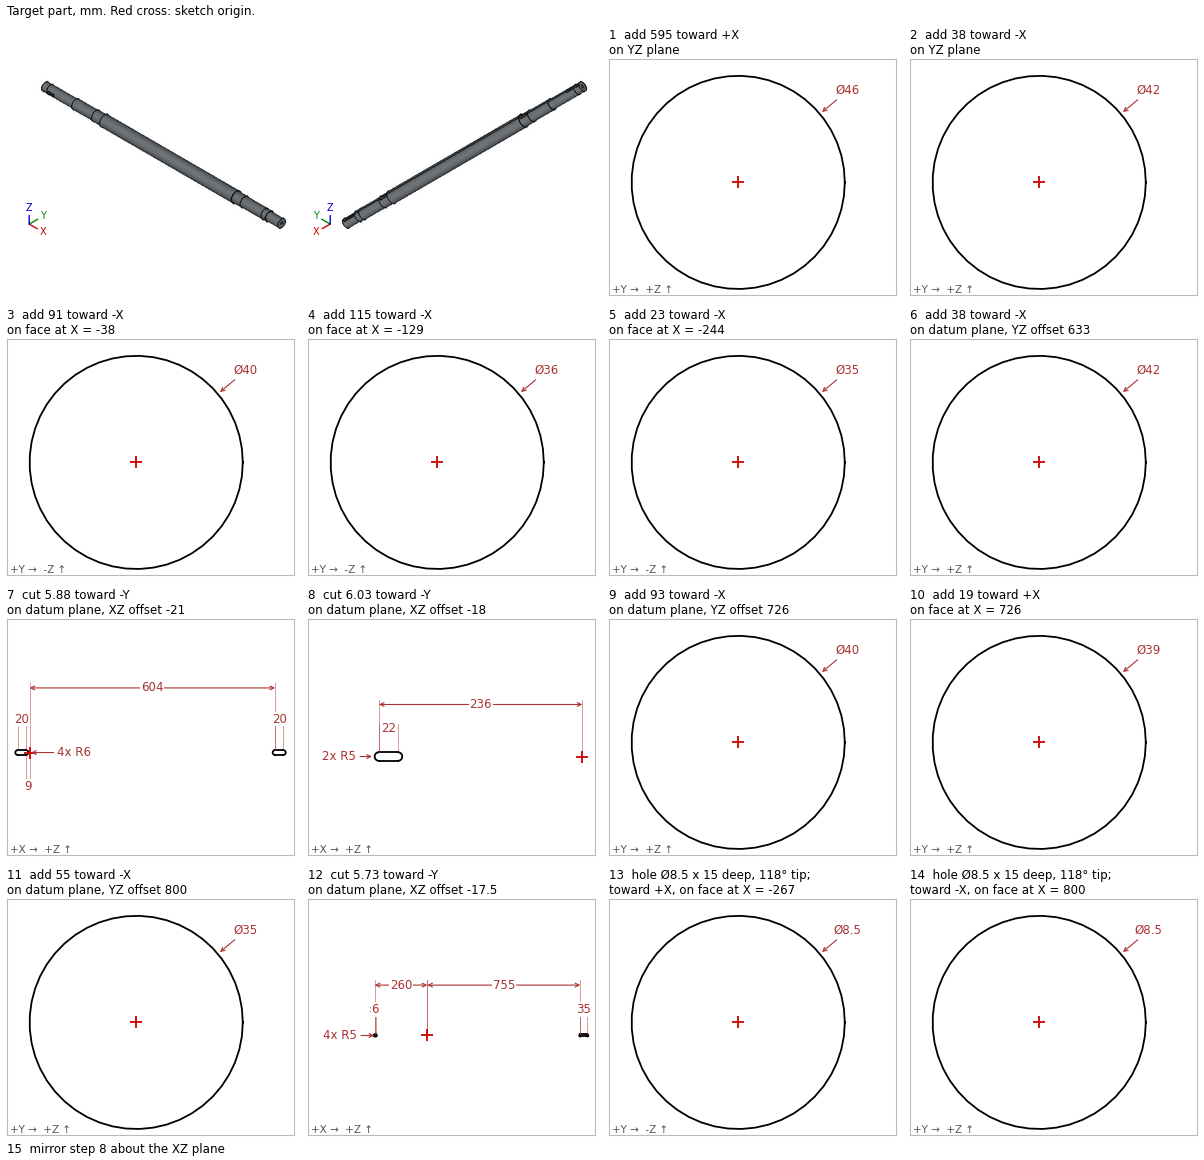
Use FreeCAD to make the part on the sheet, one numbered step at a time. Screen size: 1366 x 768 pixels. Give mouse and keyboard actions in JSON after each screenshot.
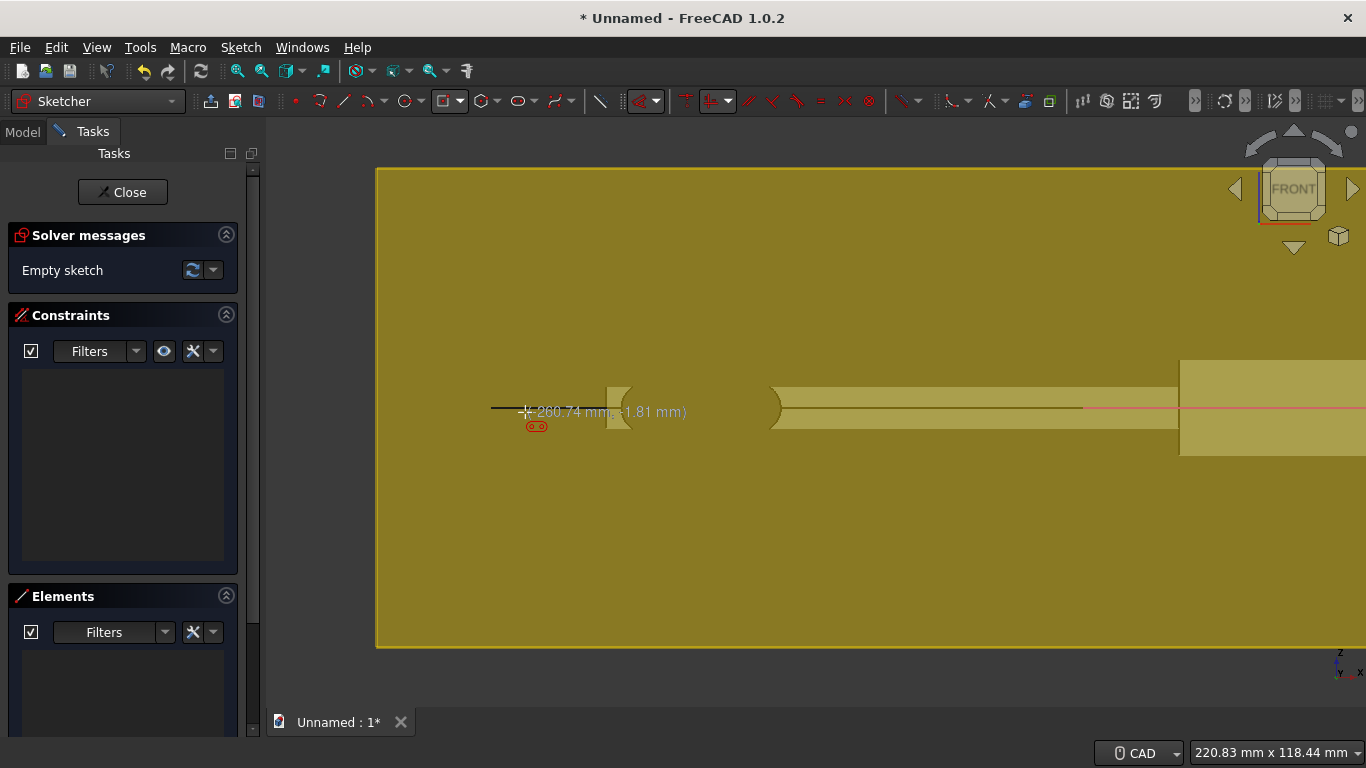
{"action": "scroll", "coordinate": [449, 413], "scroll_direction": "down", "scroll_amount": 11}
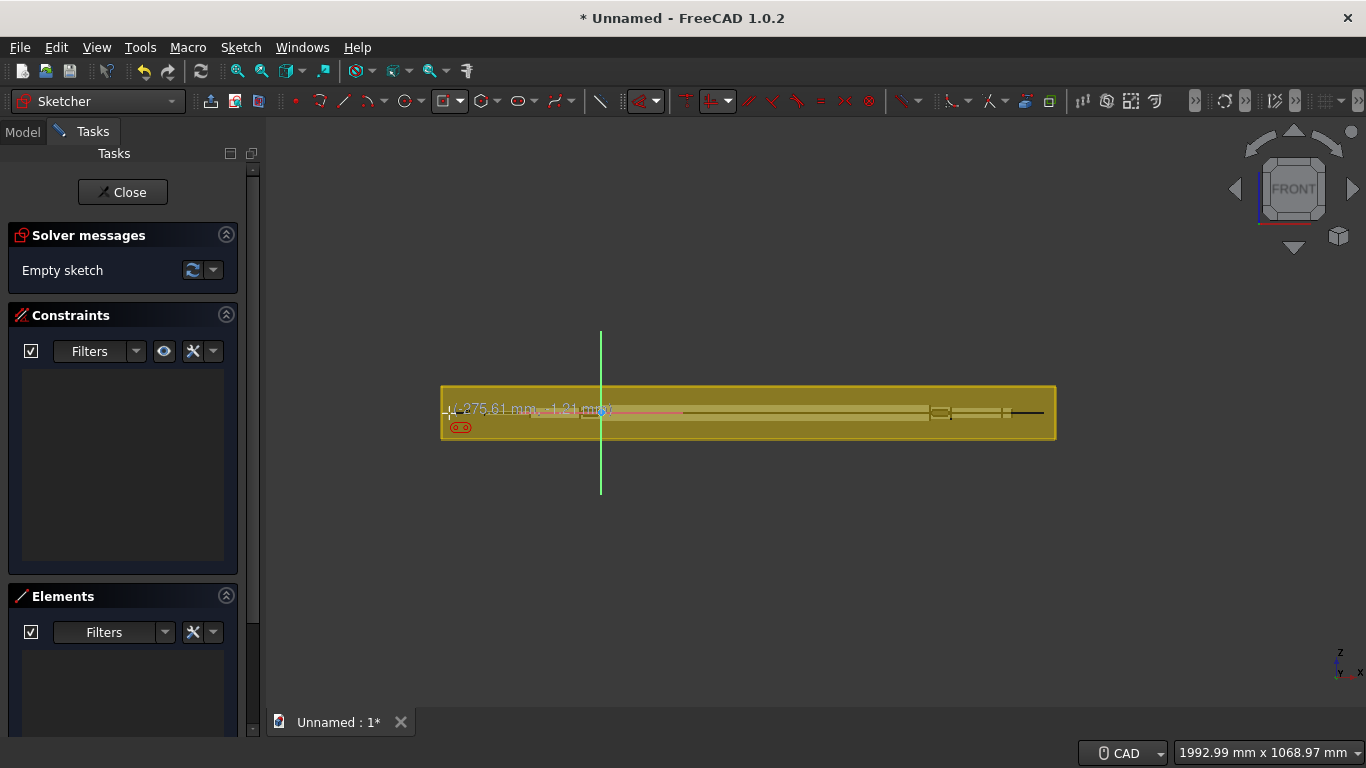
{"action": "left_click", "coordinate": [458, 413]}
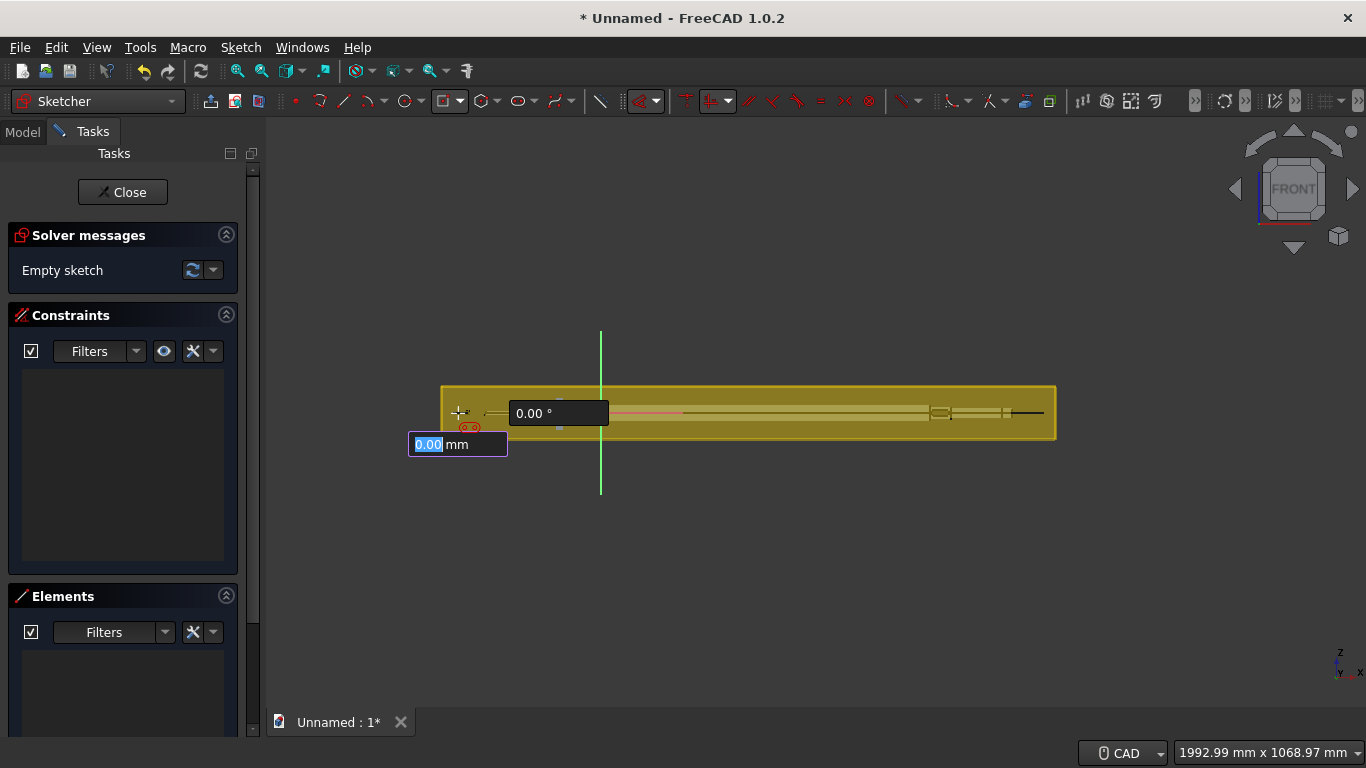
{"action": "scroll", "coordinate": [461, 413], "scroll_direction": "up", "scroll_amount": 8}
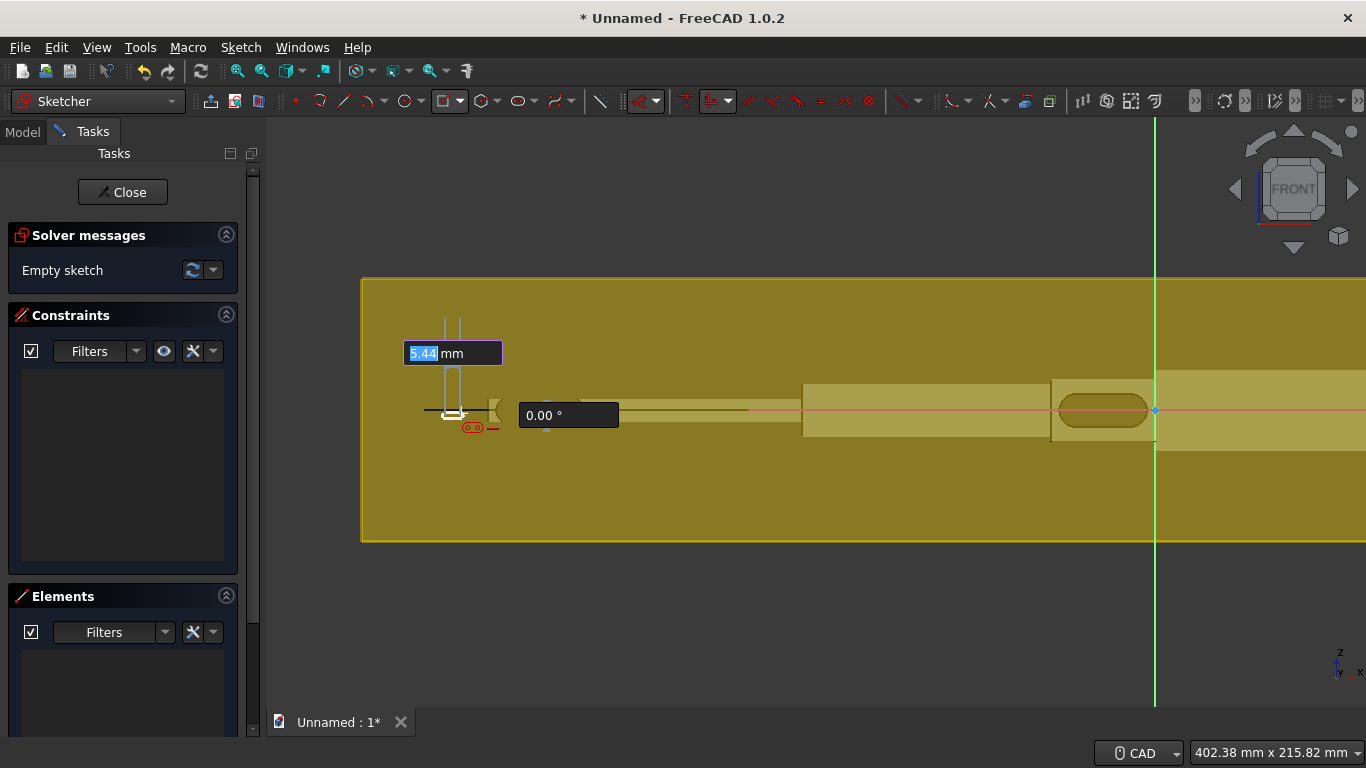
{"action": "left_click", "coordinate": [461, 401]}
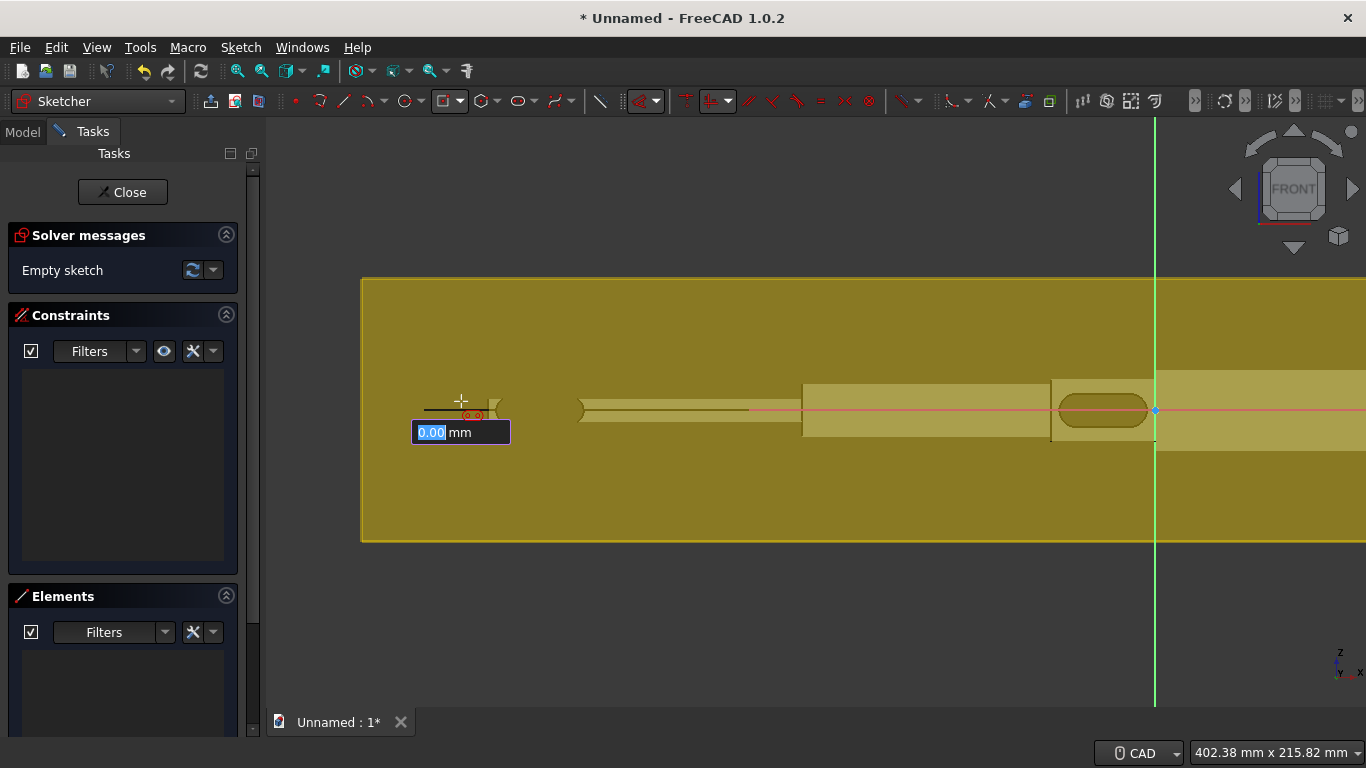
{"action": "left_click", "coordinate": [452, 397]}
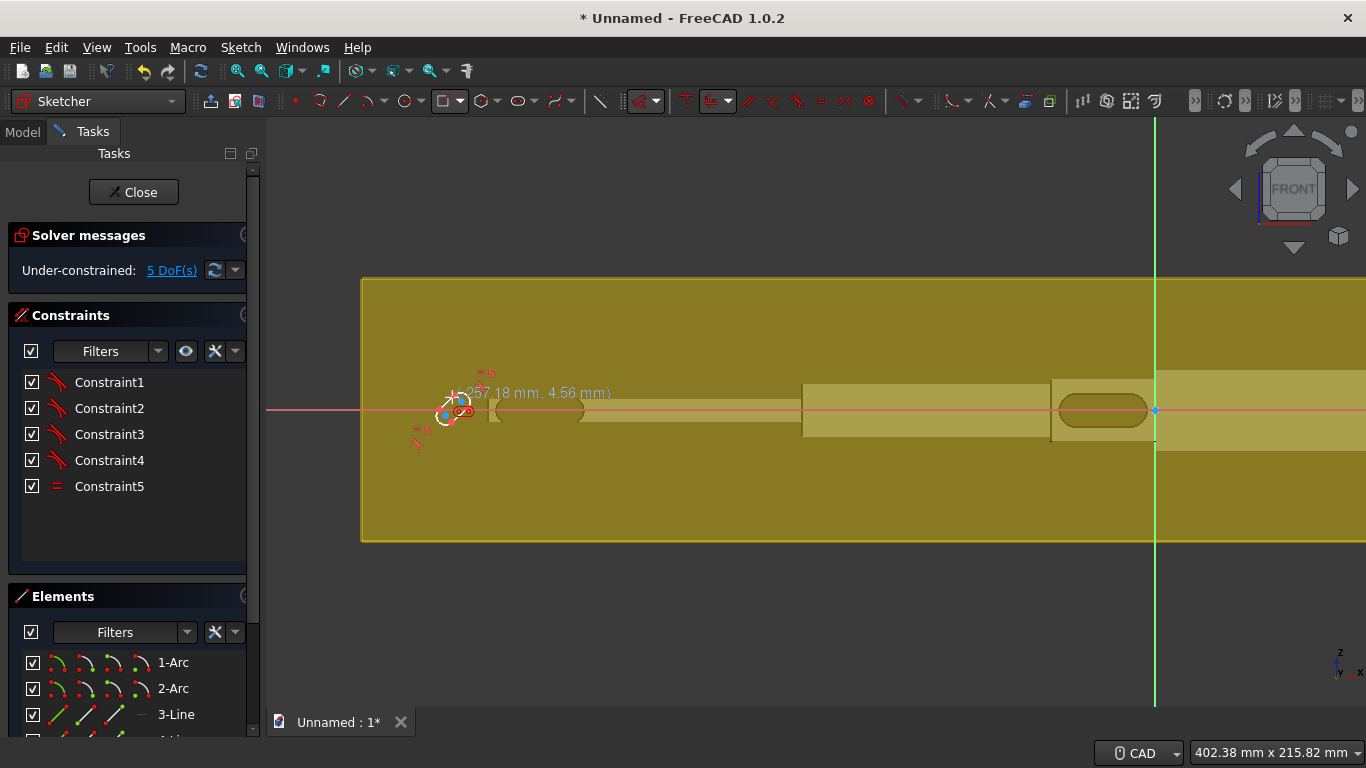
{"action": "scroll", "coordinate": [461, 412], "scroll_direction": "down", "scroll_amount": 8}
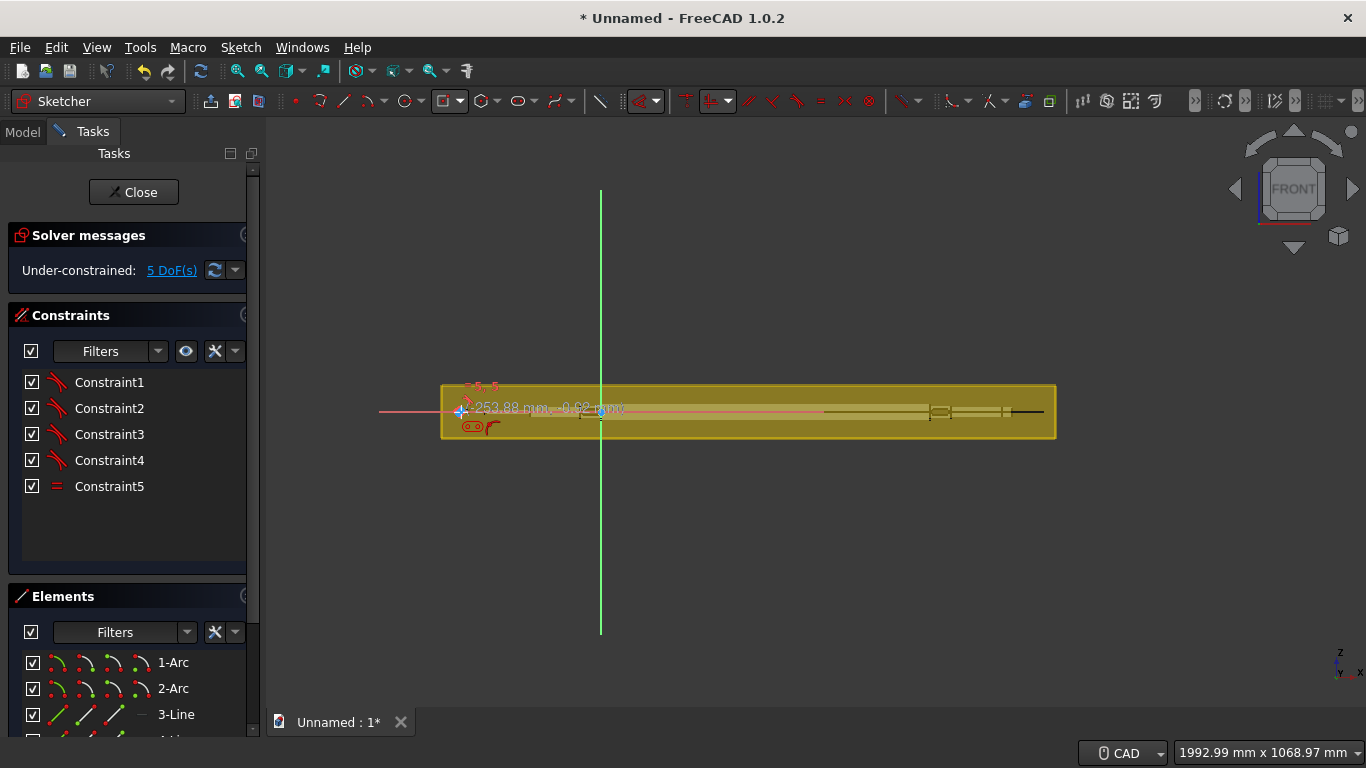
{"action": "scroll", "coordinate": [1018, 412], "scroll_direction": "up", "scroll_amount": 11}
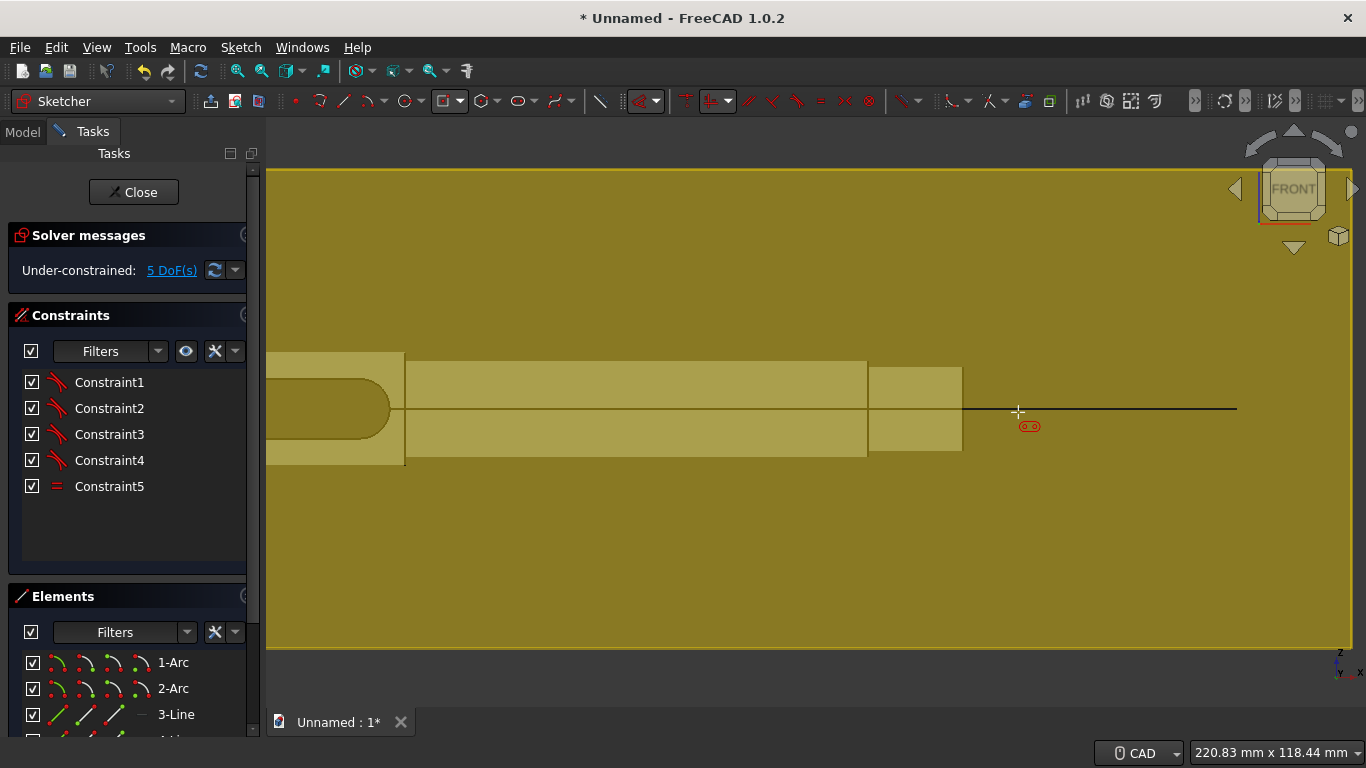
{"action": "scroll", "coordinate": [1019, 412], "scroll_direction": "down", "scroll_amount": 11}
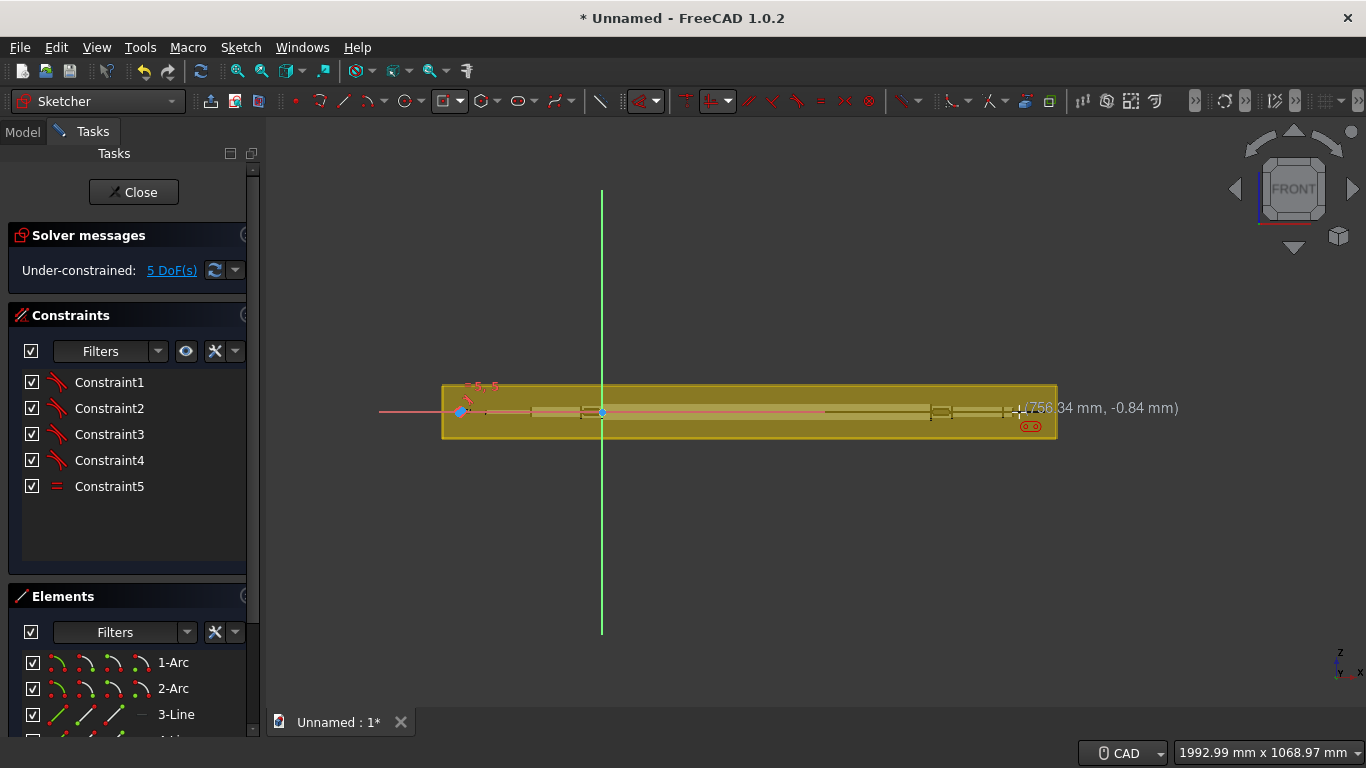
{"action": "left_click", "coordinate": [1019, 412]}